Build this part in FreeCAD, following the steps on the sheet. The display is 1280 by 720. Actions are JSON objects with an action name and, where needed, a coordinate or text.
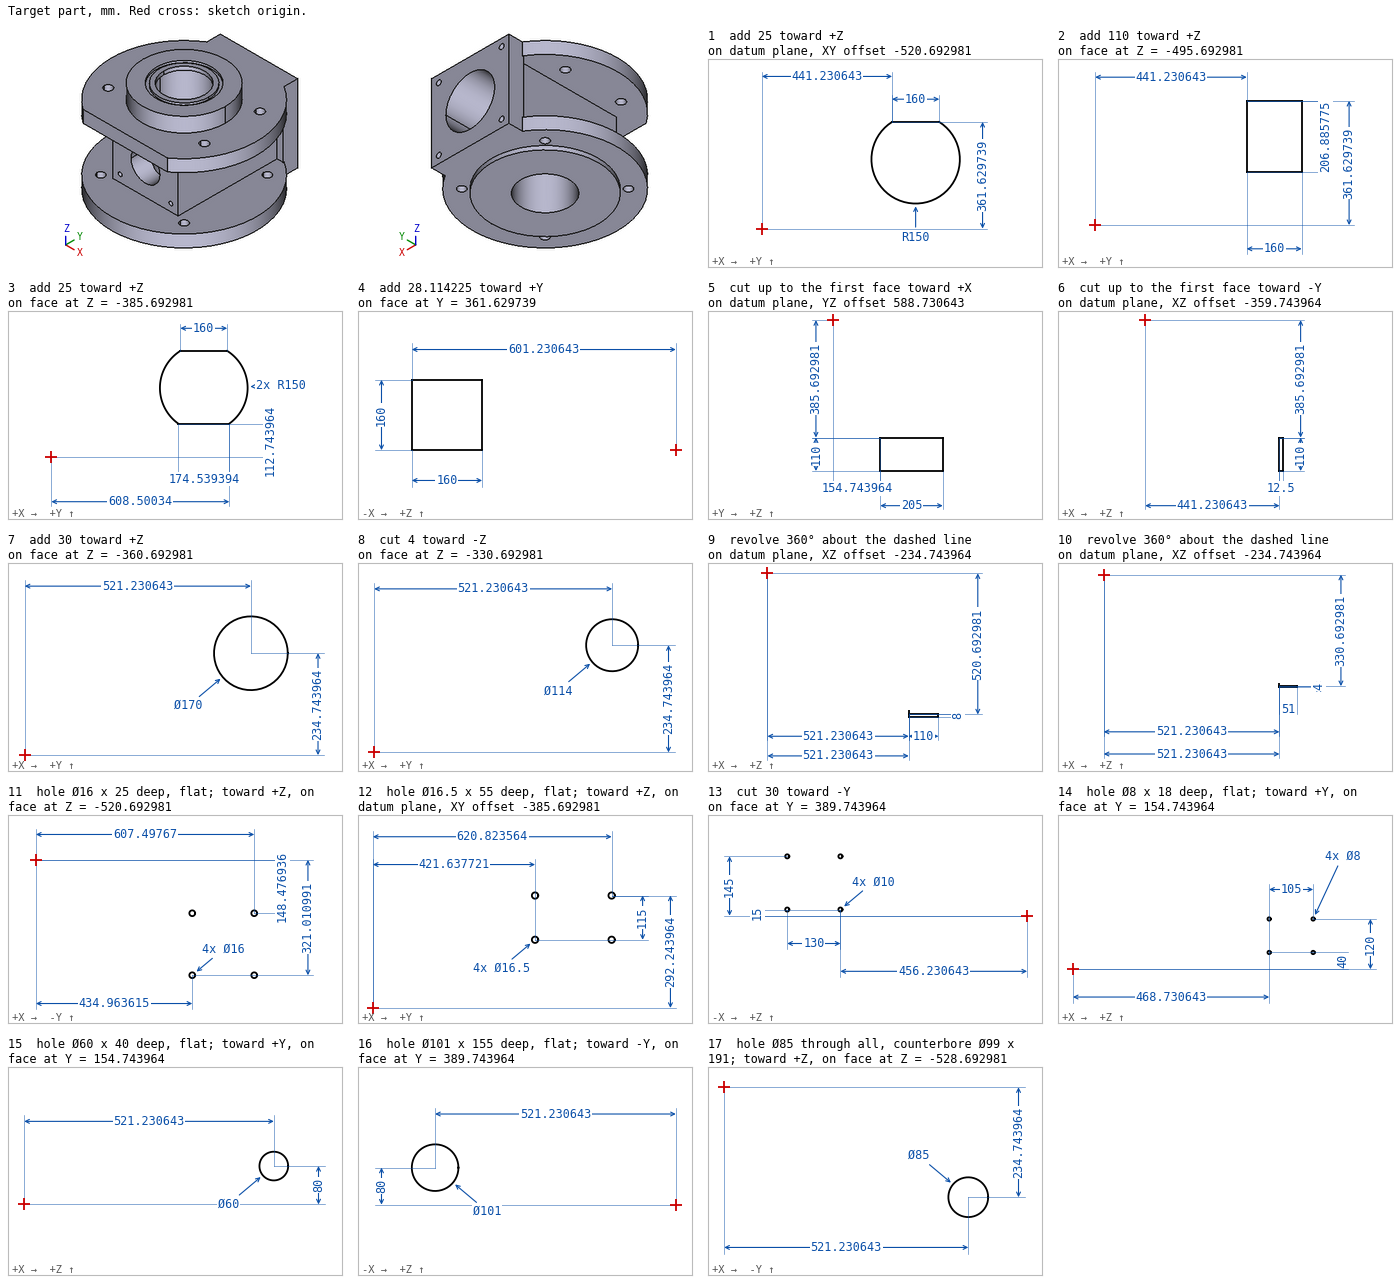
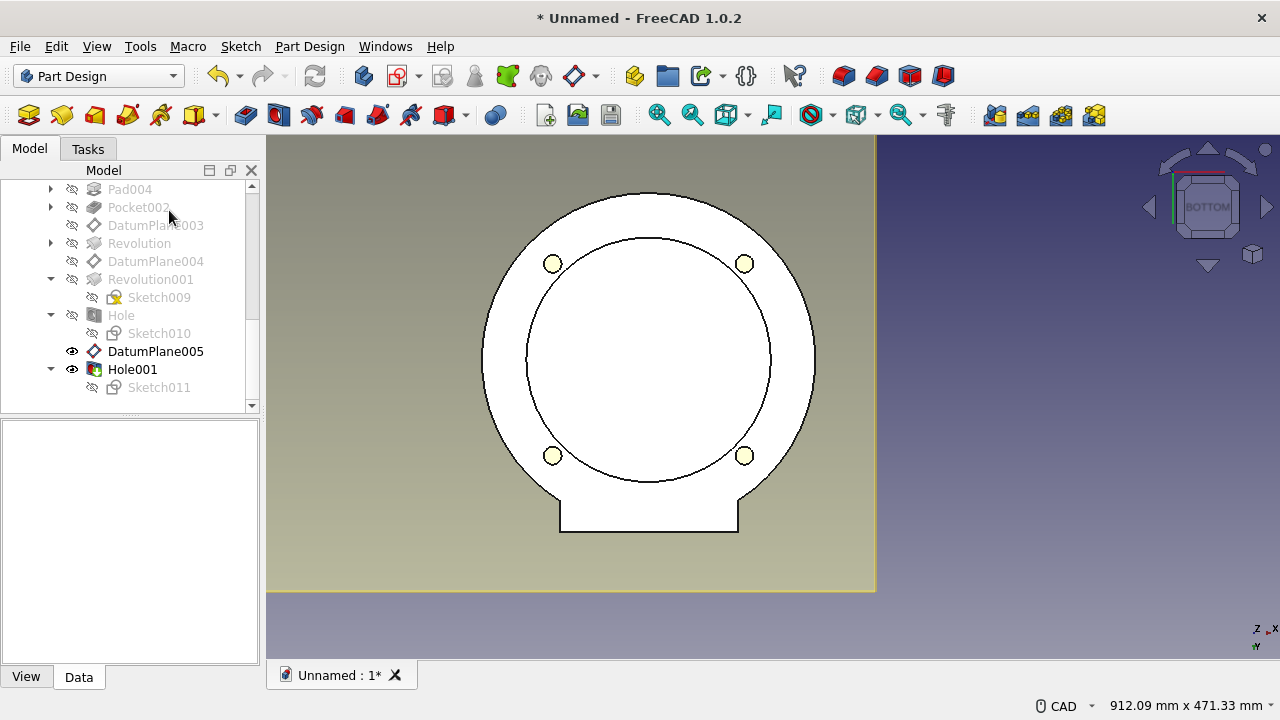
{"action": "left_click", "coordinate": [117, 351]}
{"action": "key", "text": "space"}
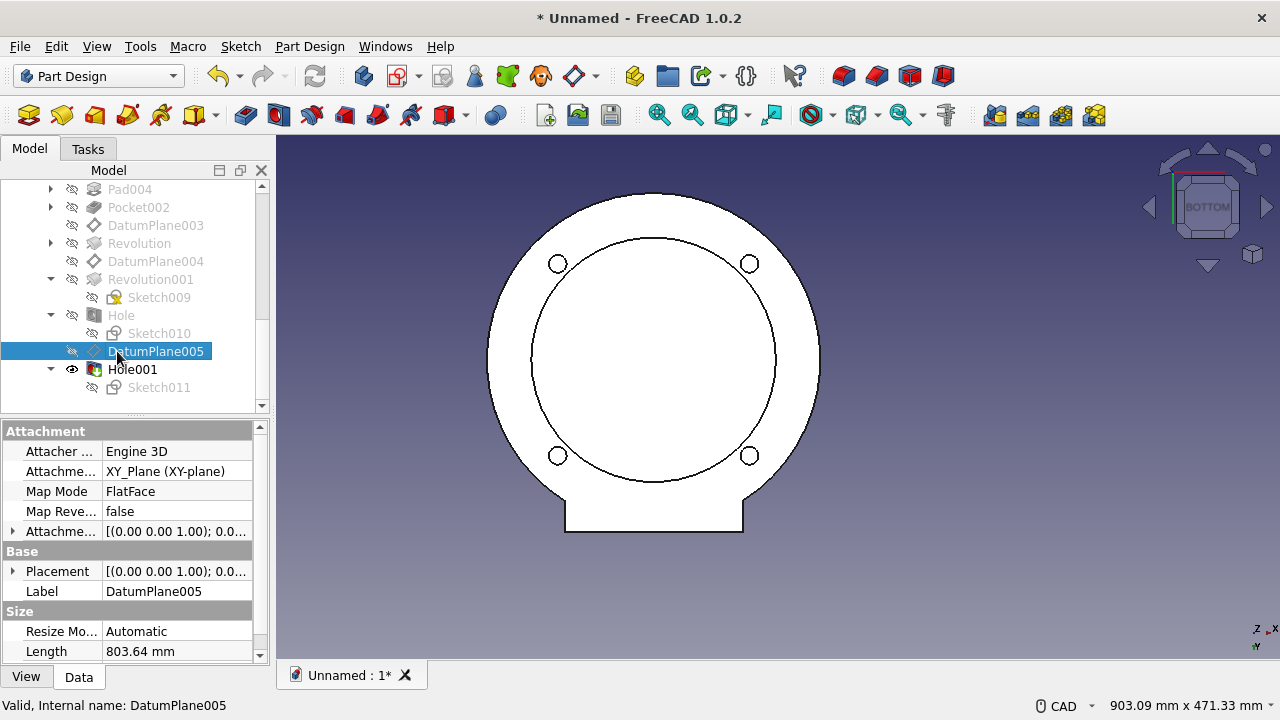
{"action": "key", "text": "4"}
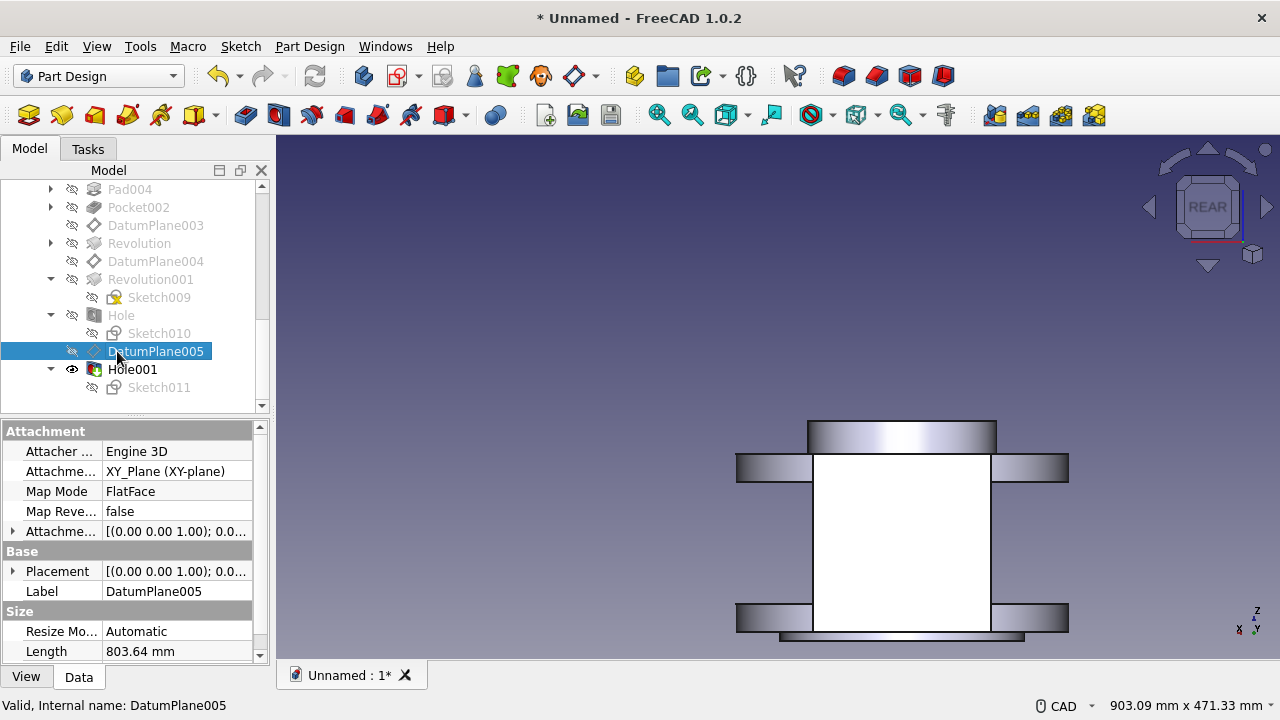
{"action": "left_click", "coordinate": [660, 116]}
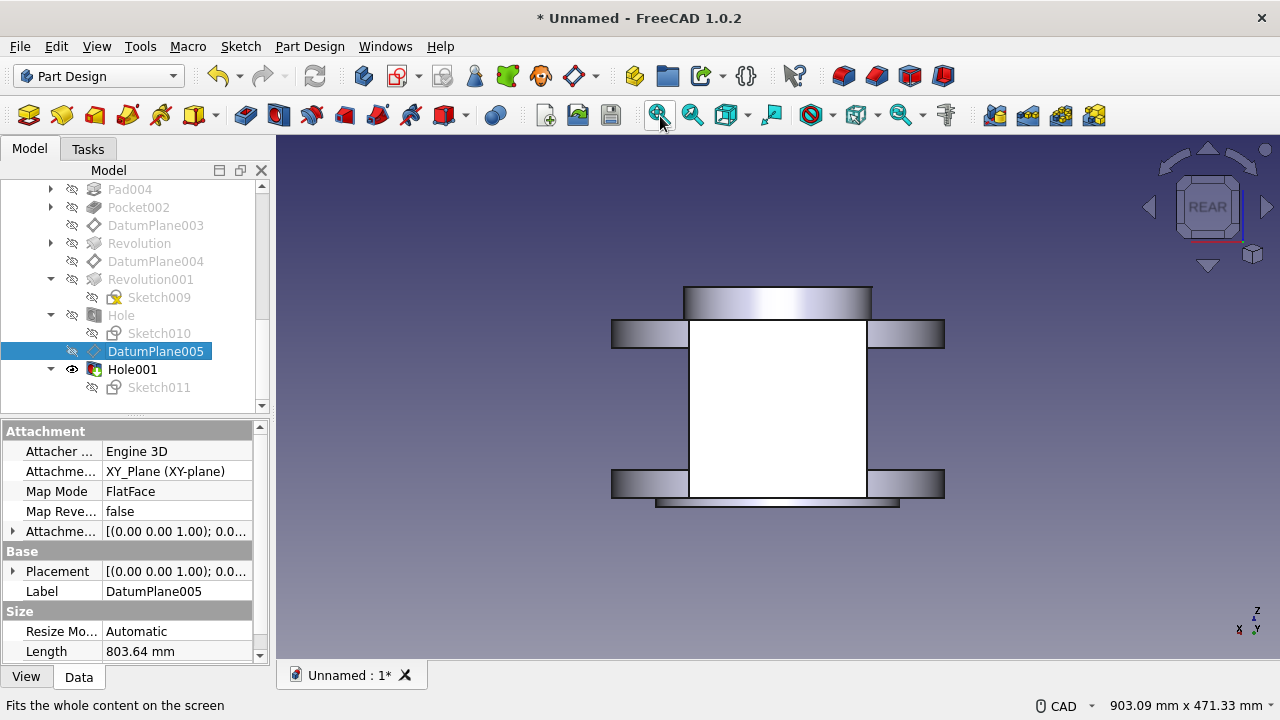
{"action": "left_click", "coordinate": [778, 408]}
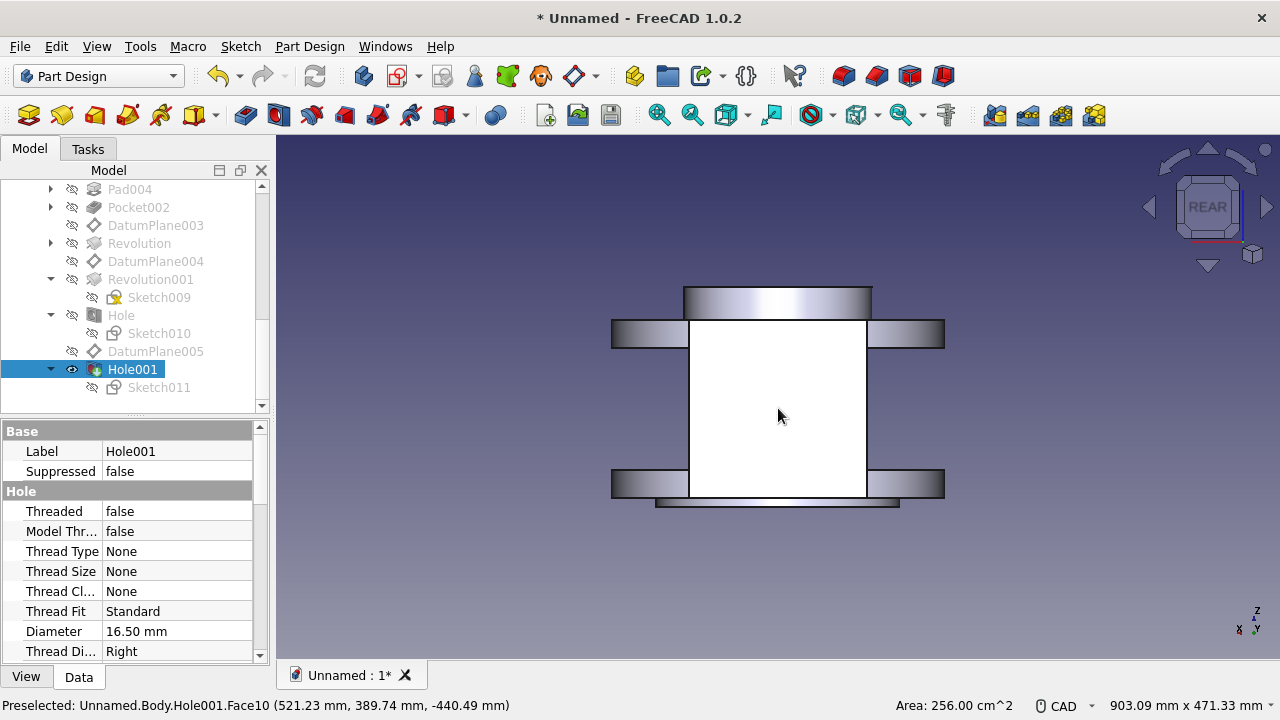
{"action": "left_click", "coordinate": [396, 76]}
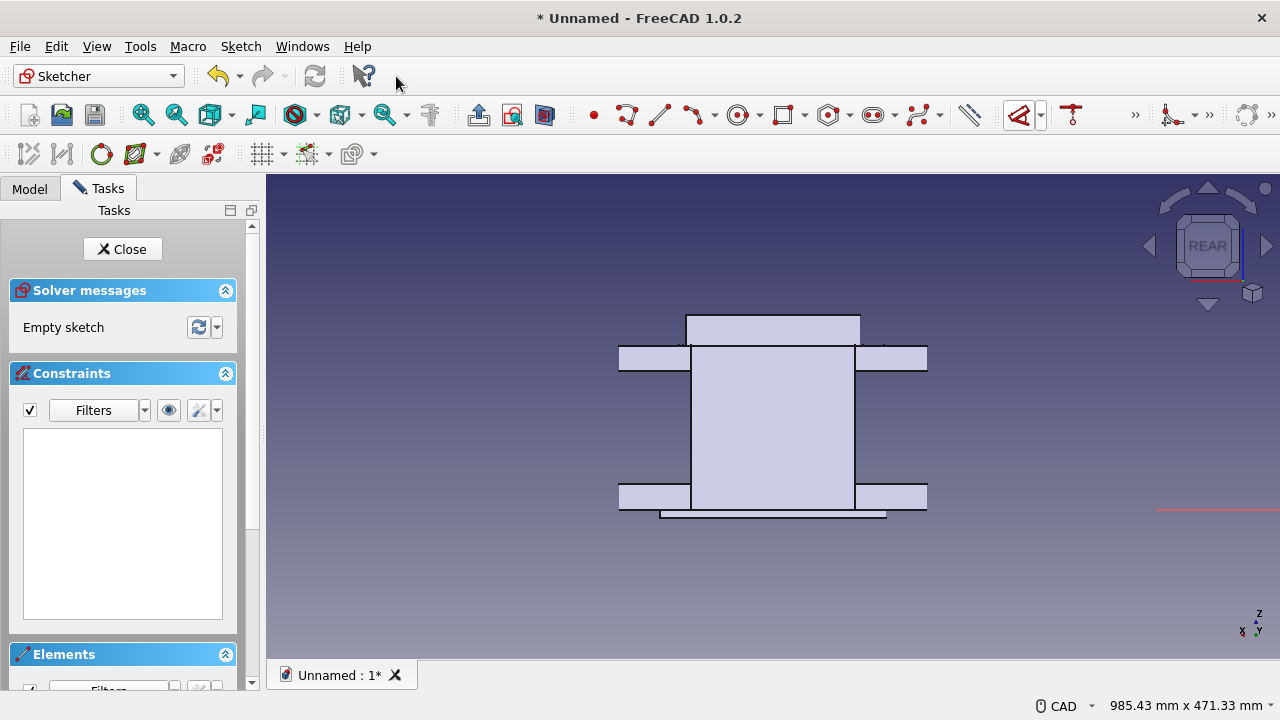
{"action": "scroll", "coordinate": [829, 437], "scroll_direction": "up", "scroll_amount": 4}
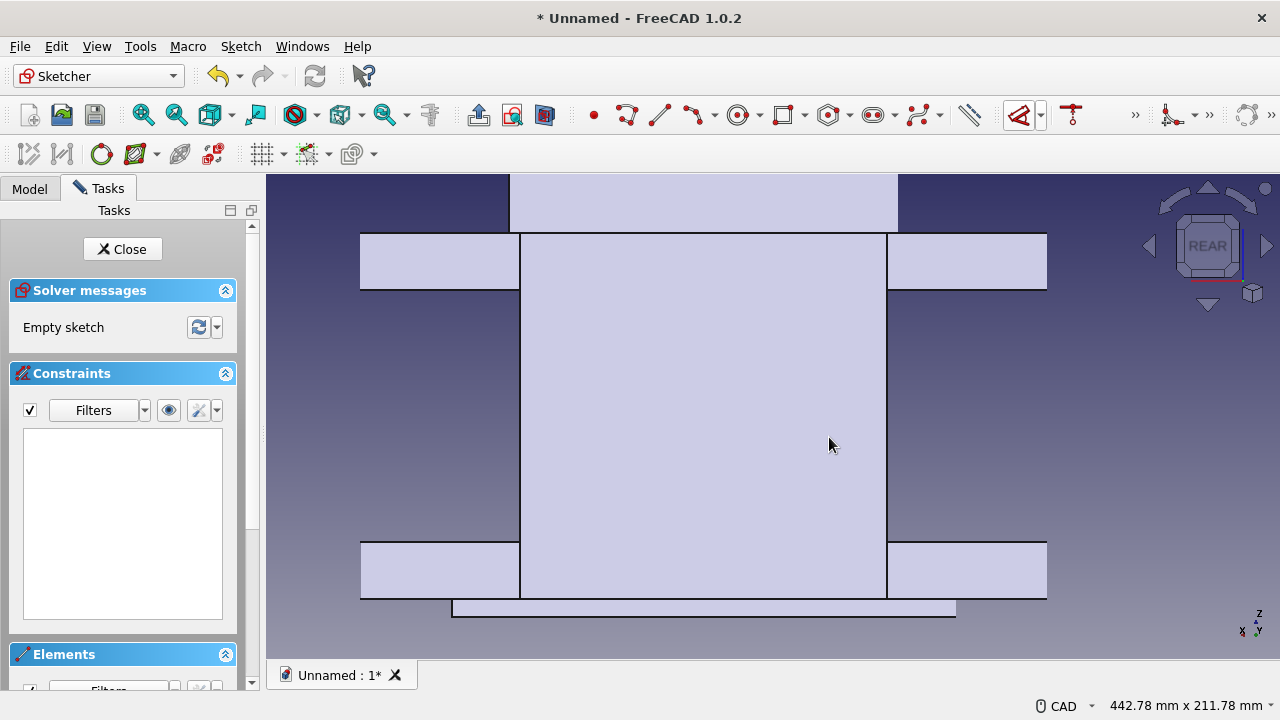
{"action": "left_click", "coordinate": [738, 116]}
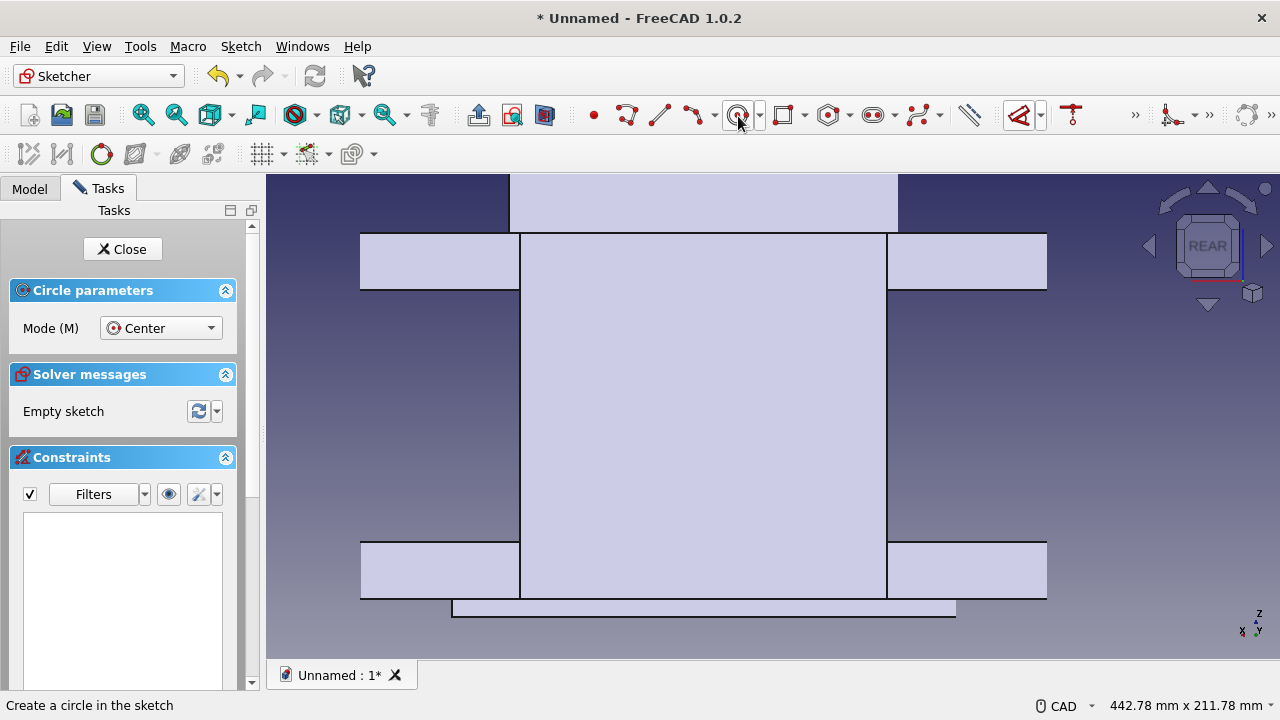
{"action": "scroll", "coordinate": [853, 565], "scroll_direction": "up", "scroll_amount": 4}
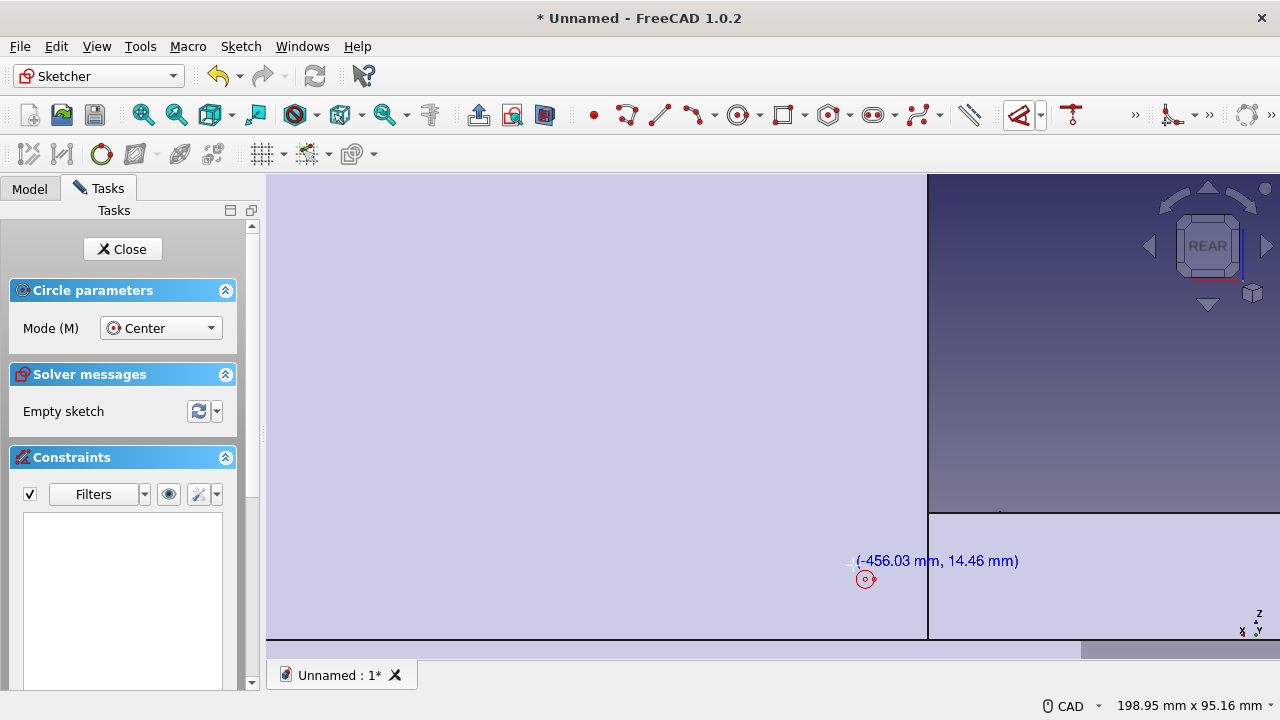
{"action": "left_click", "coordinate": [851, 563]}
{"action": "left_click", "coordinate": [869, 545]}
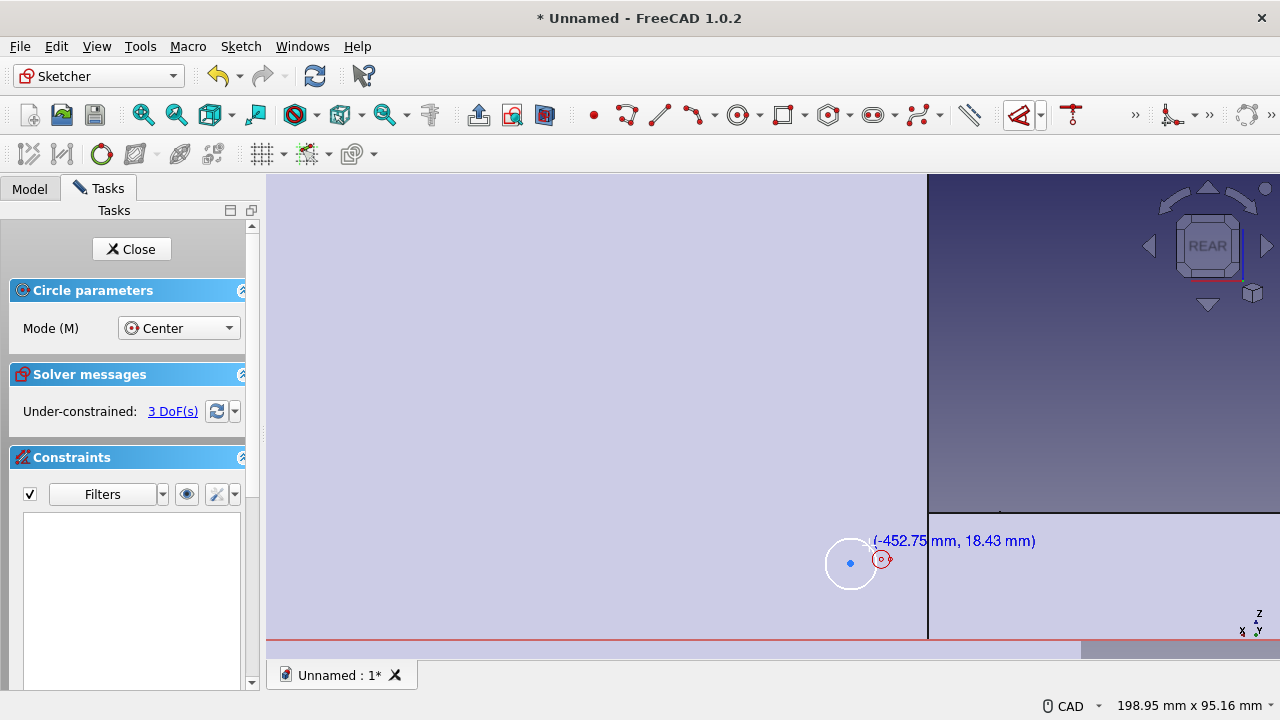
{"action": "scroll", "coordinate": [855, 567], "scroll_direction": "down", "scroll_amount": 4}